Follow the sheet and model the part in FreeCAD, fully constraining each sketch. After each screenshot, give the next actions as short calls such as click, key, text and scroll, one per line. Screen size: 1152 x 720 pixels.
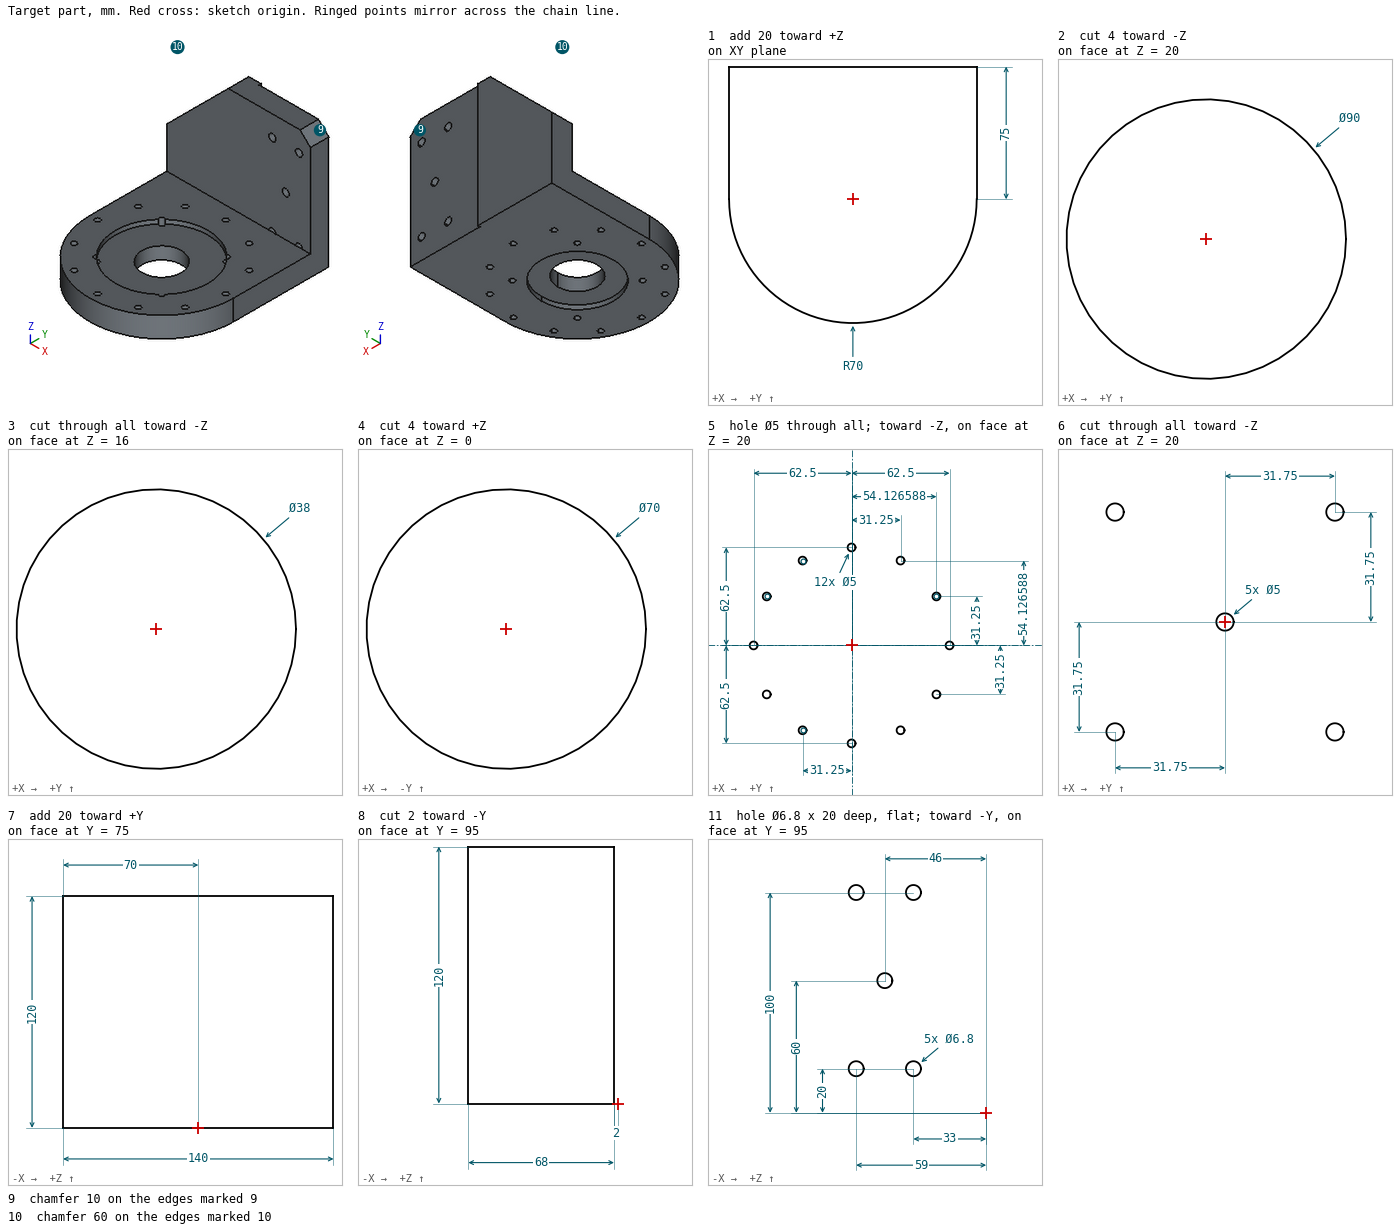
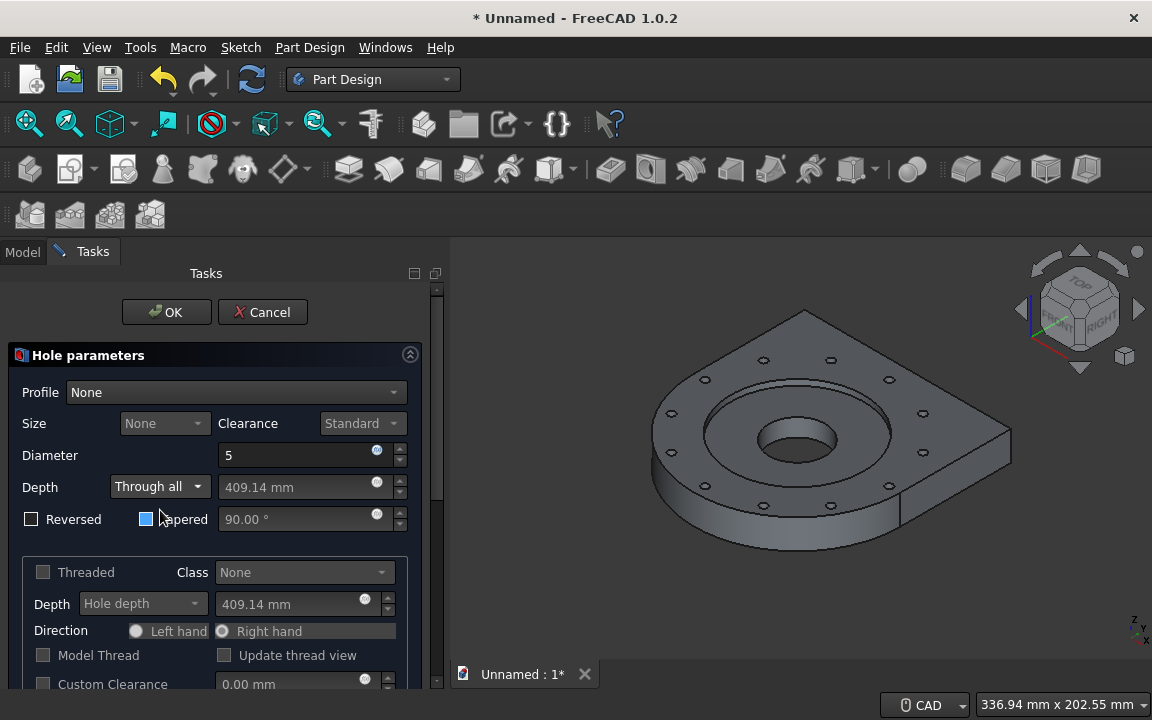
click(167, 312)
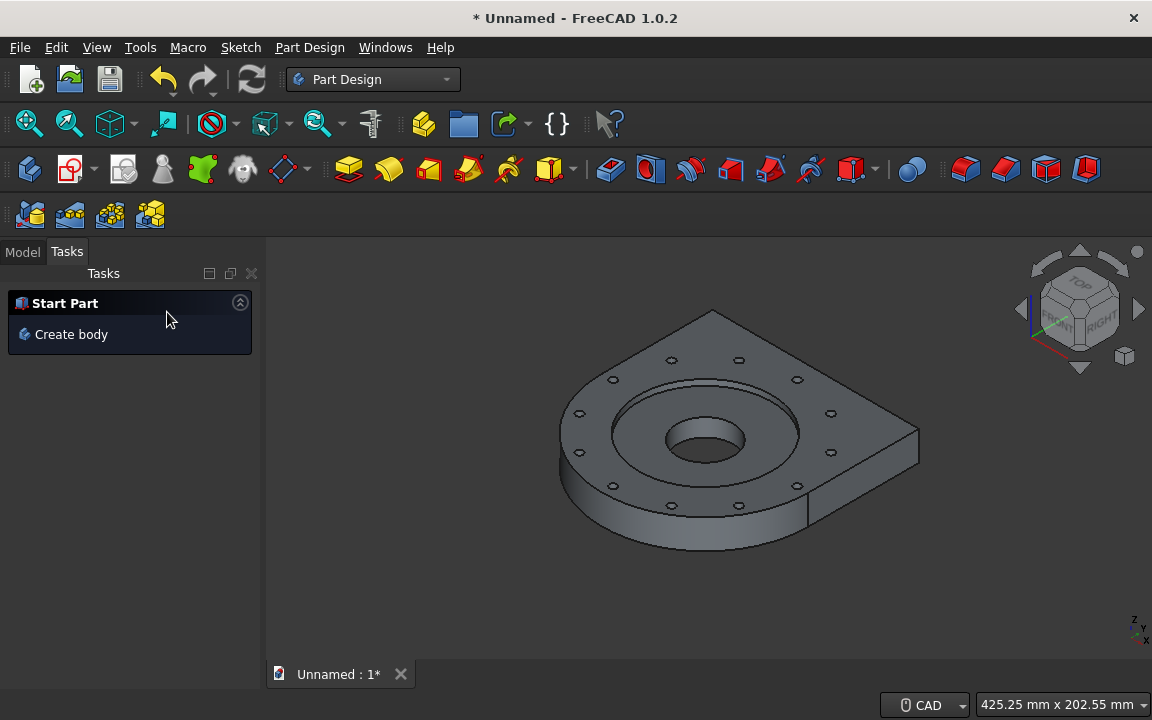
click(711, 361)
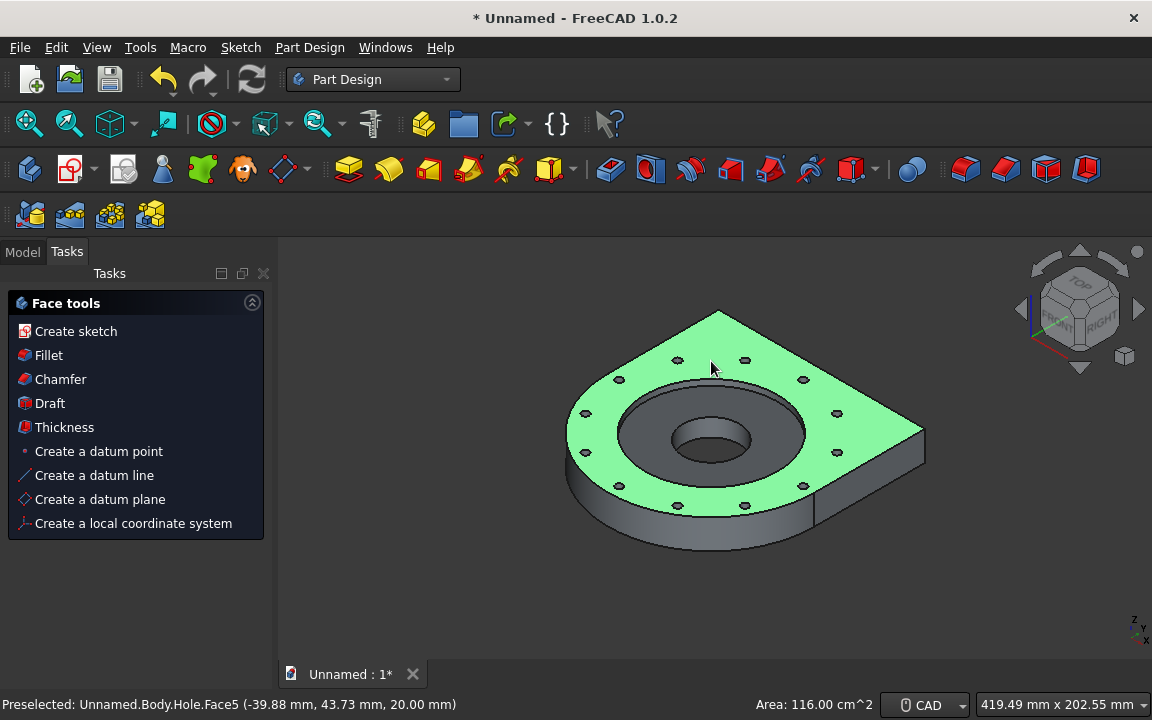
click(70, 170)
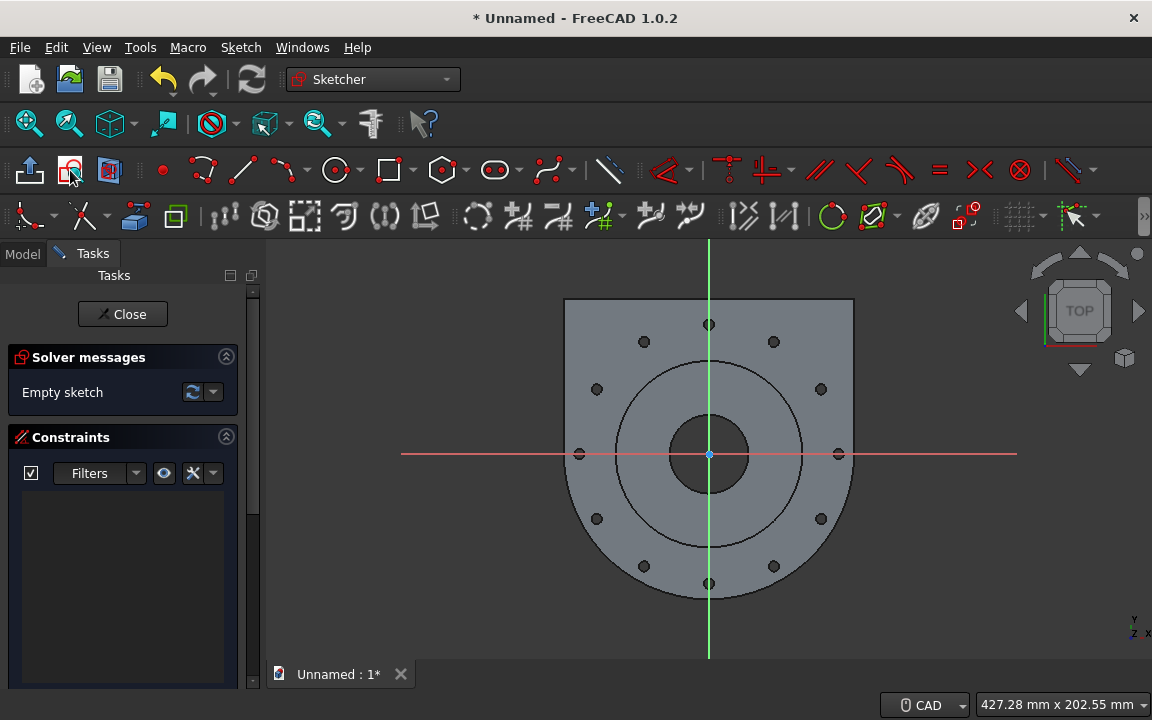
scroll(792, 460, up, 3)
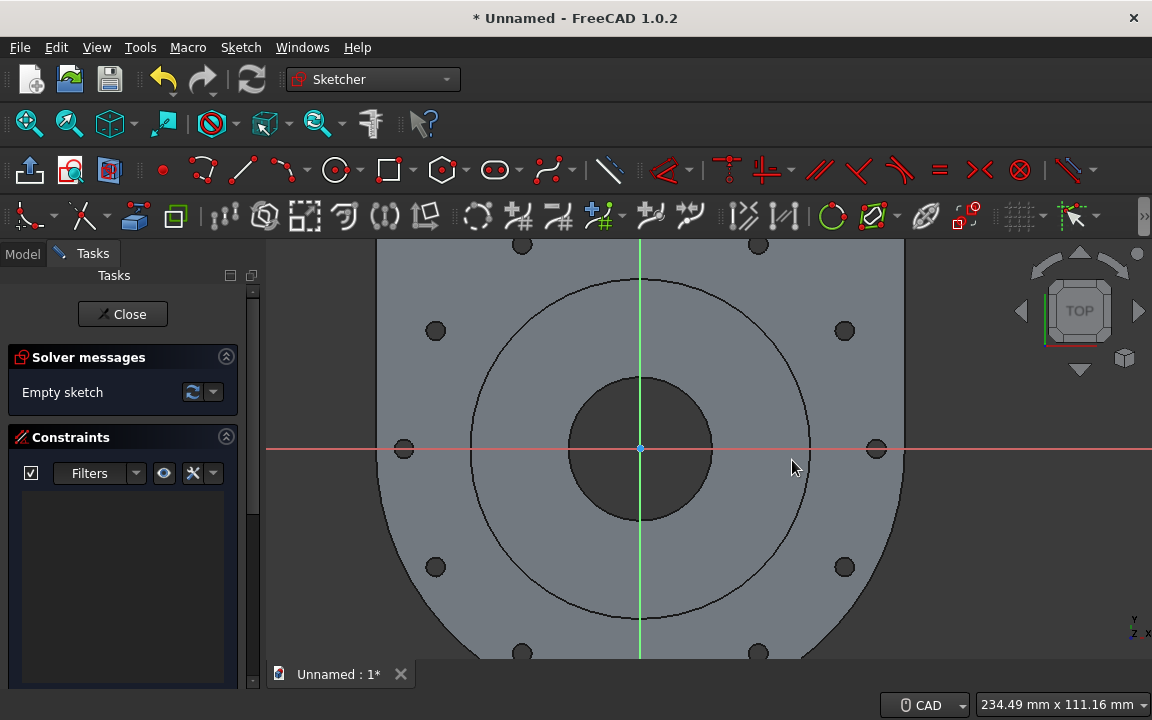
key(g)
key(c)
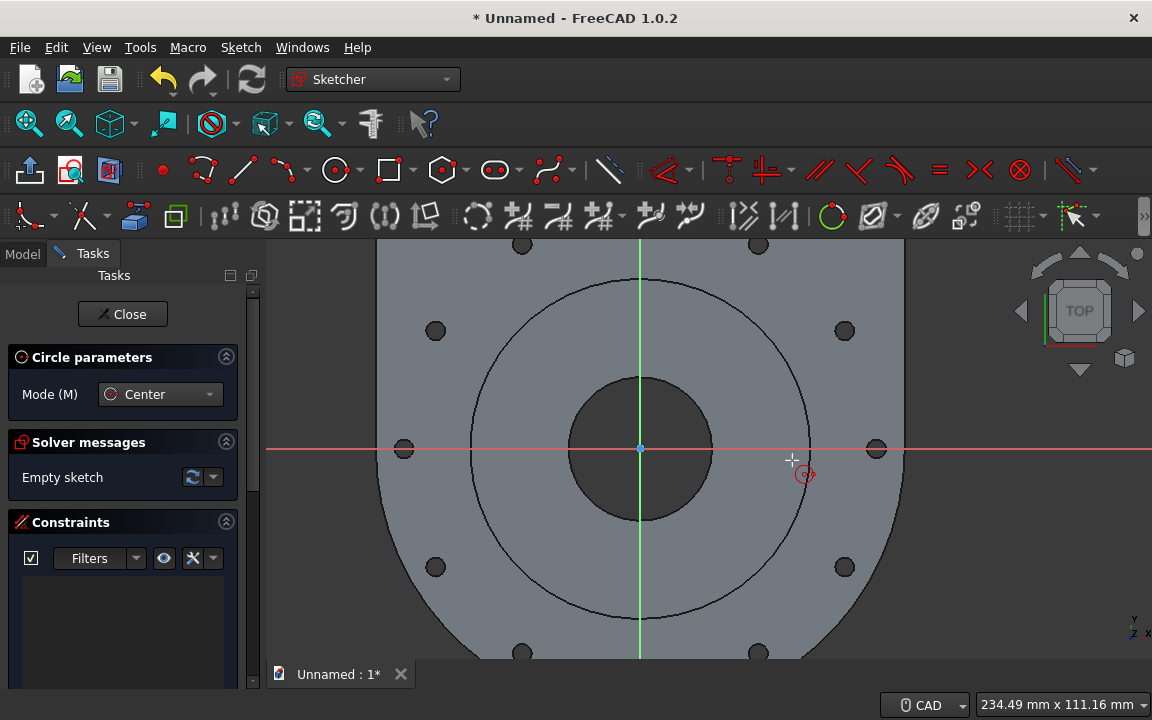
scroll(640, 449, up, 5)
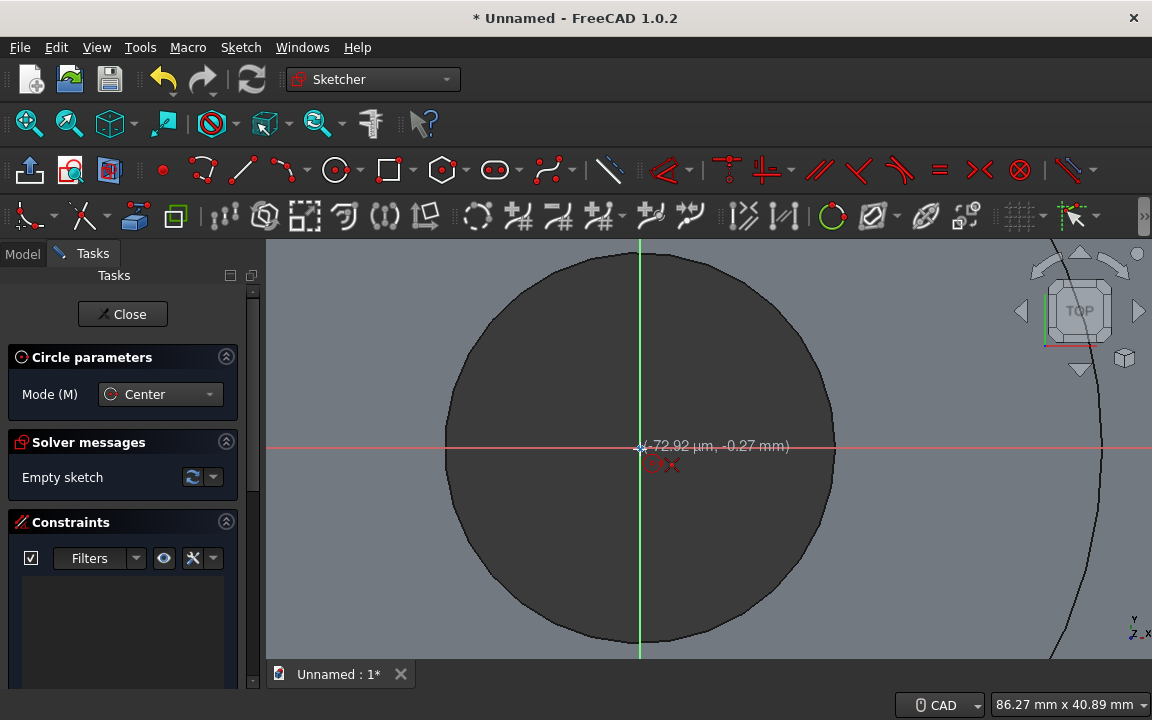
click(640, 448)
move(658, 430)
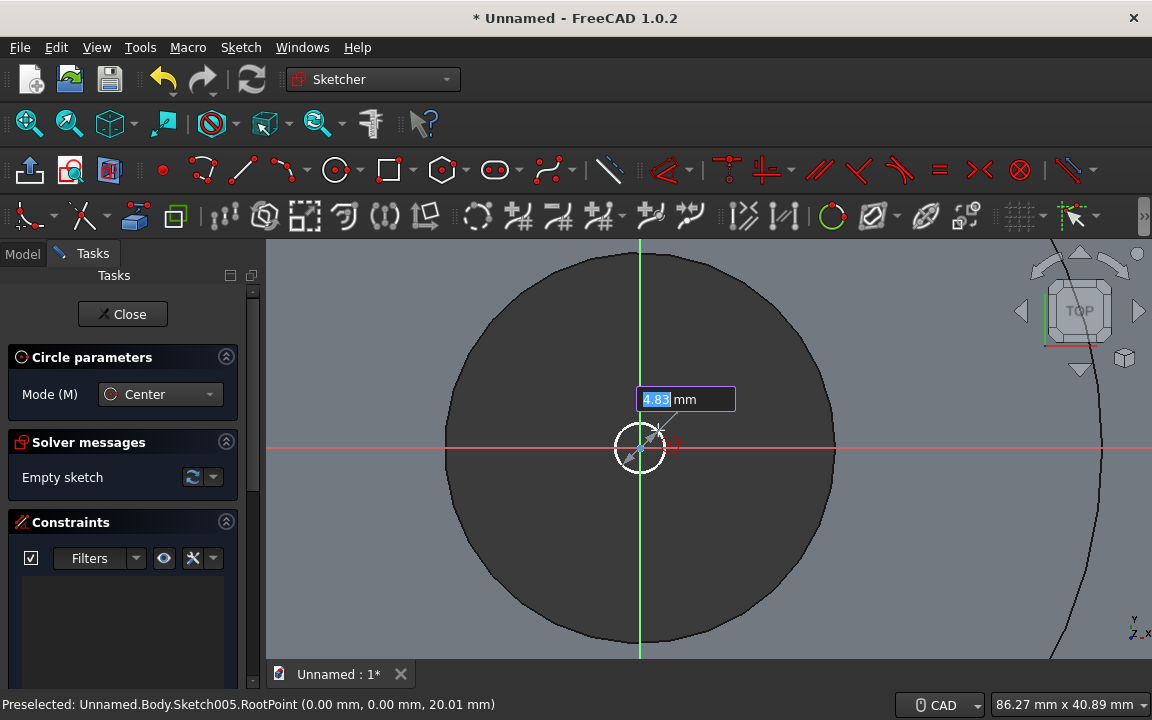
text(5)
key(Return)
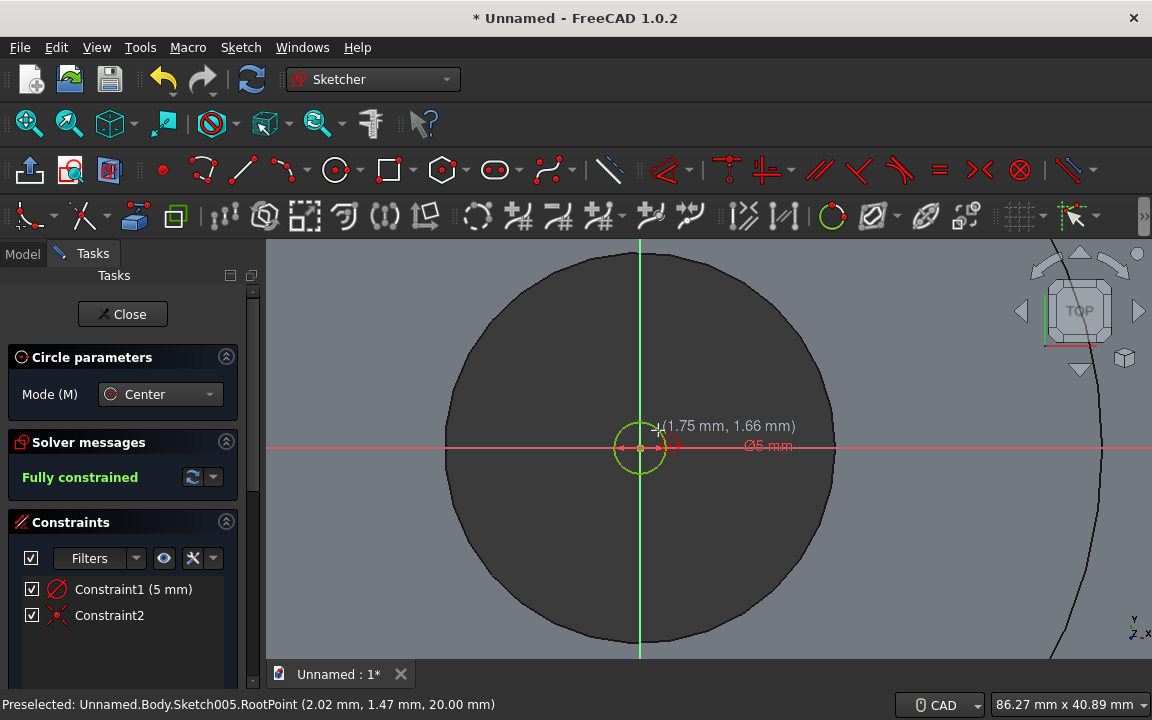
scroll(641, 450, down, 5)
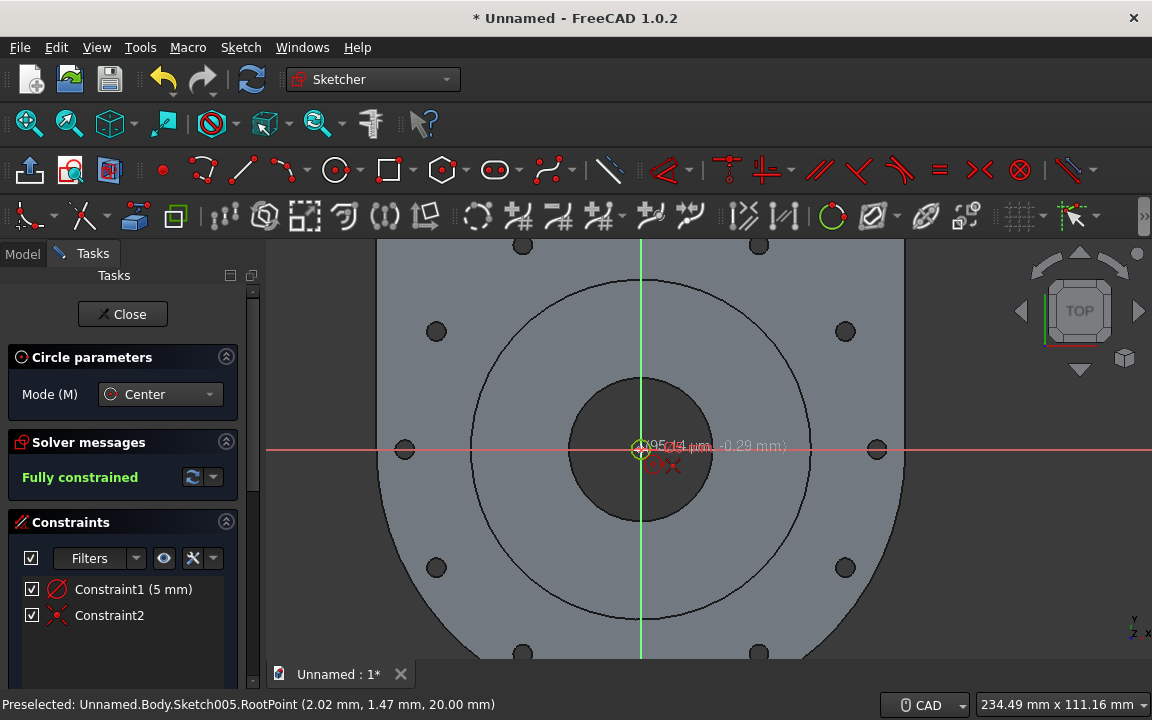
scroll(761, 330, up, 5)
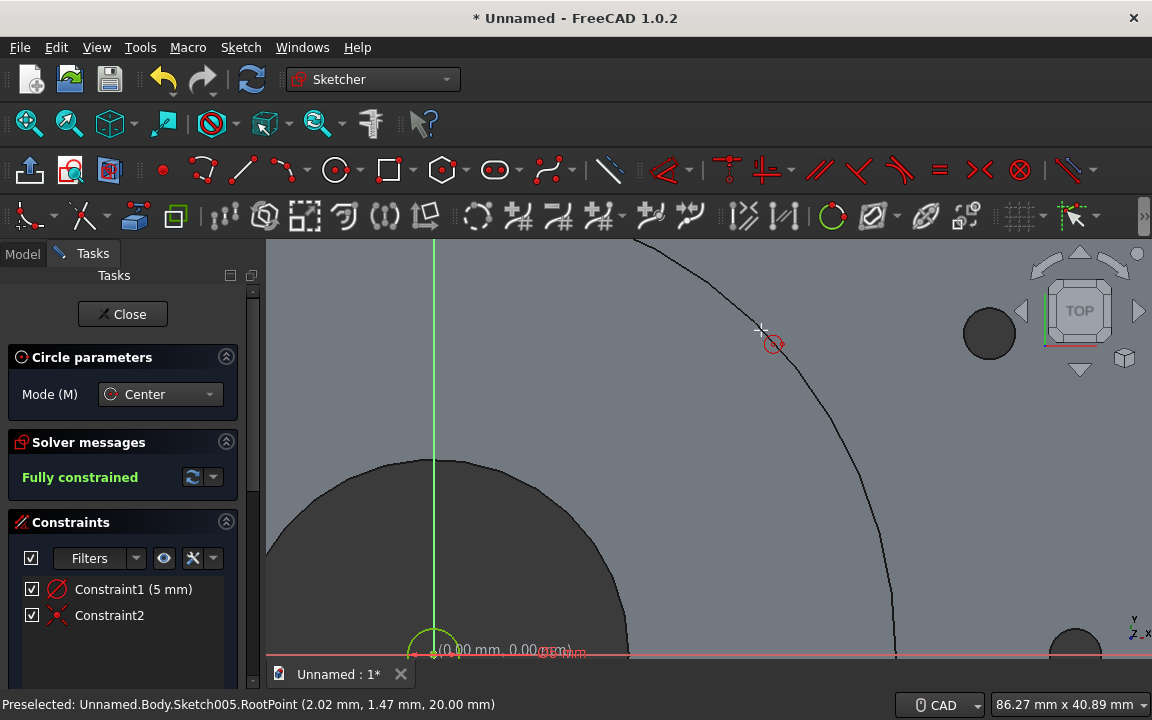
click(760, 329)
move(778, 310)